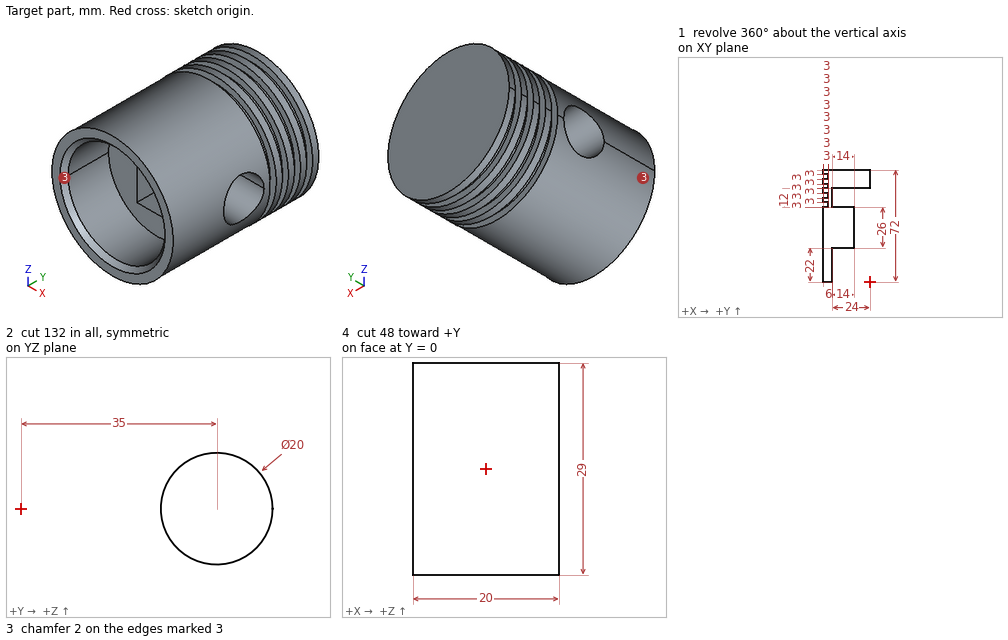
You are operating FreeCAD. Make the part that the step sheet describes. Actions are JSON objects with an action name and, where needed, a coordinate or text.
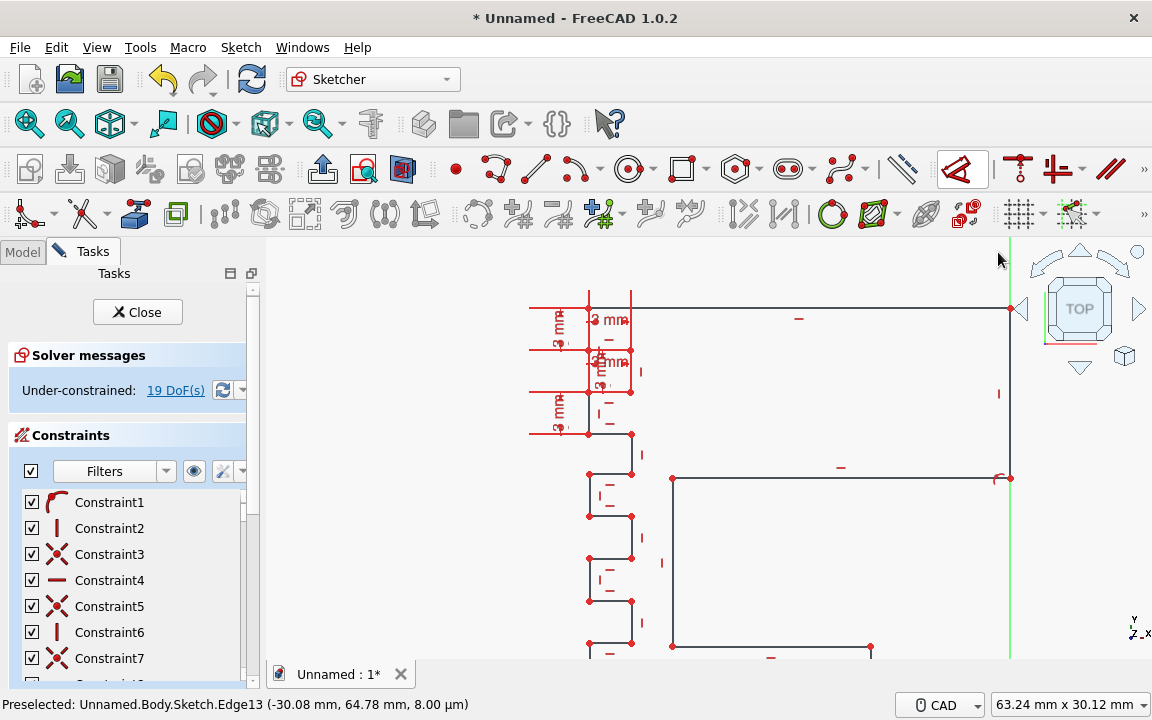
{"action": "left_click", "coordinate": [602, 434]}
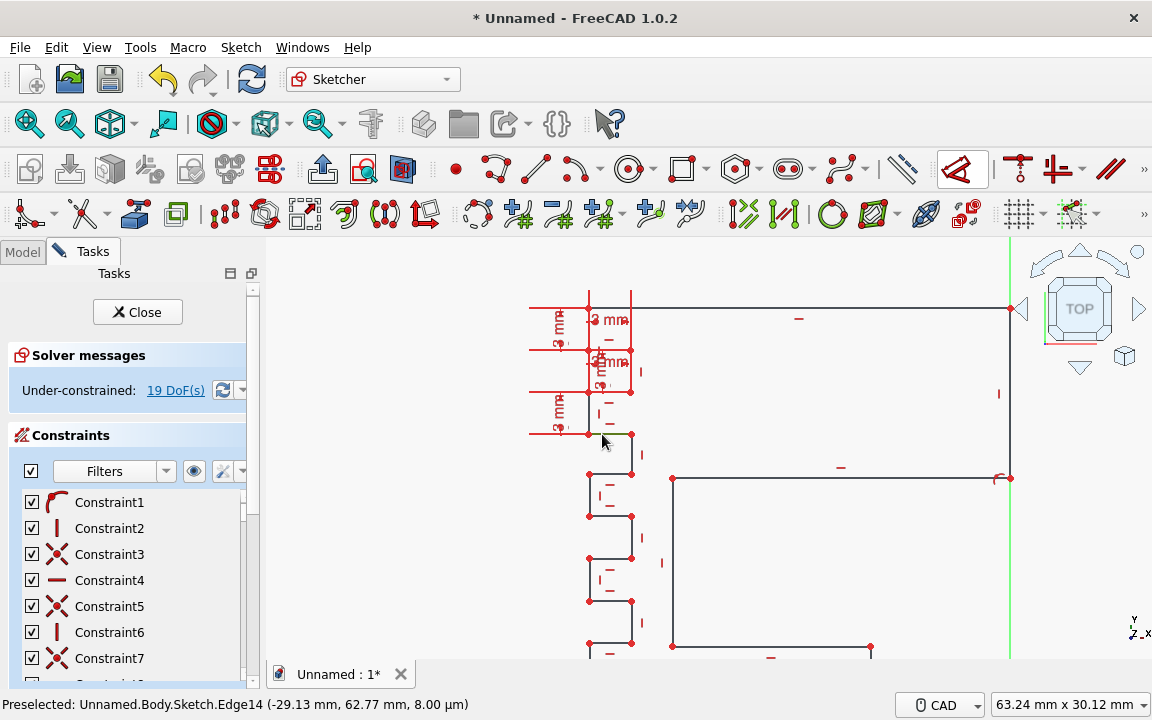
{"action": "left_click", "coordinate": [982, 170]}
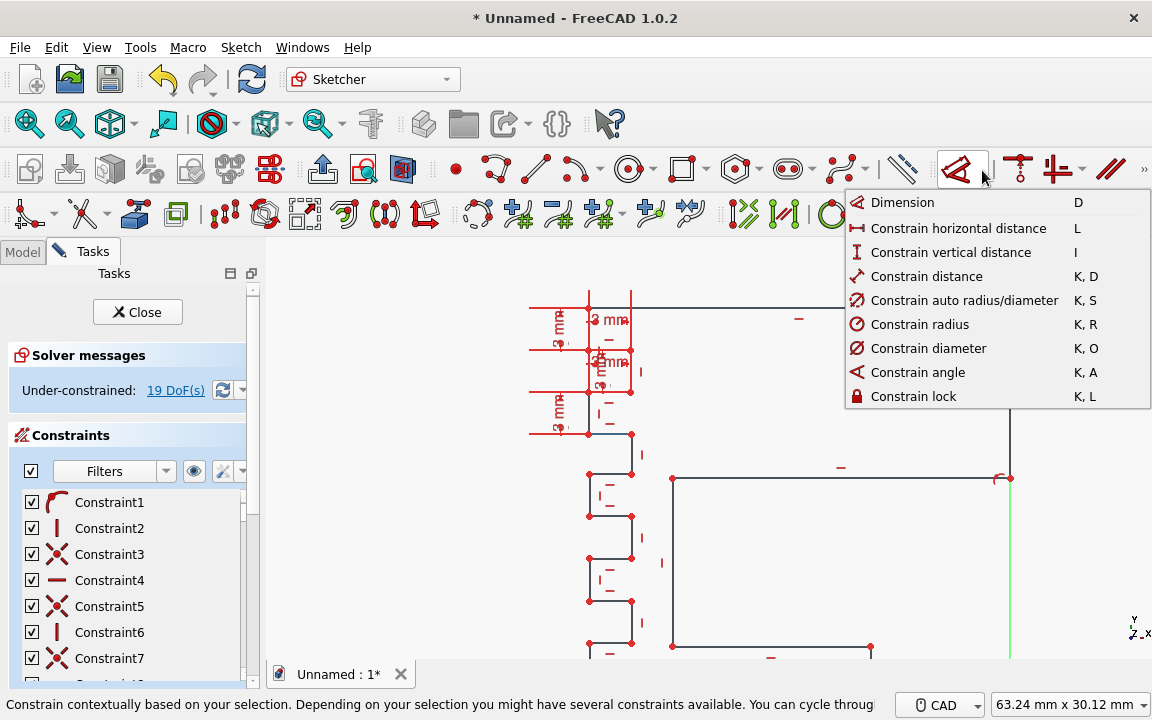
{"action": "left_click", "coordinate": [998, 228]}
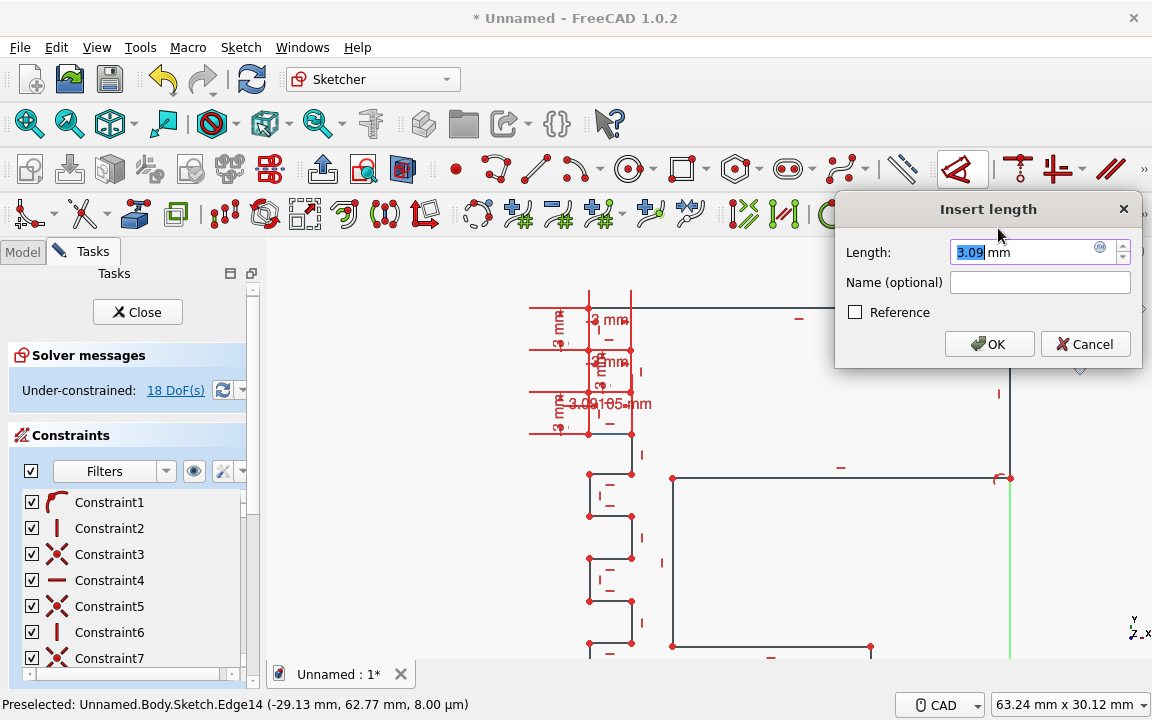
{"action": "type", "text": "3"}
{"action": "key", "text": "Return"}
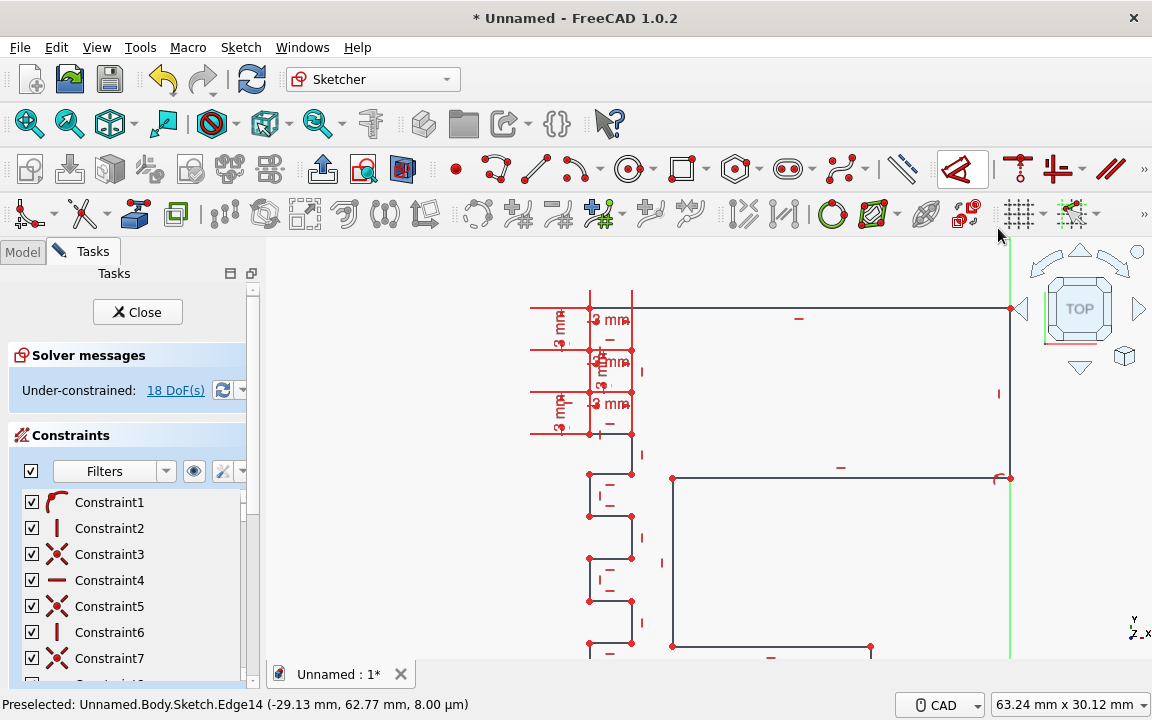
{"action": "left_click", "coordinate": [632, 446]}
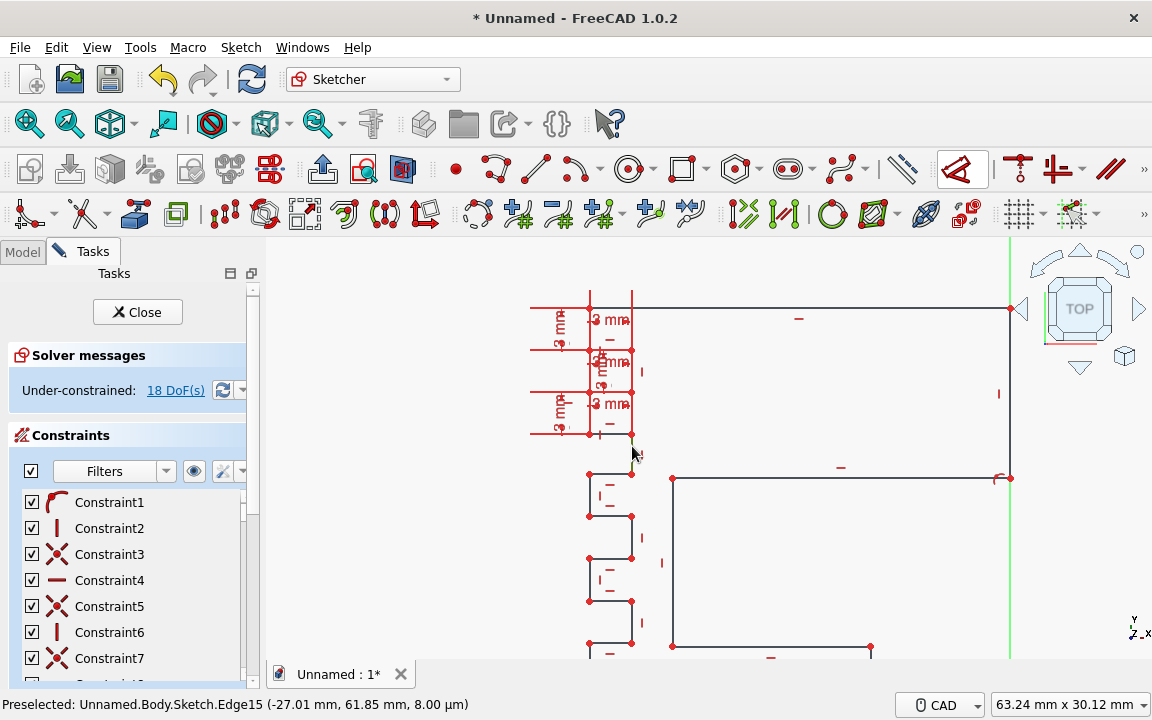
{"action": "left_click", "coordinate": [982, 170]}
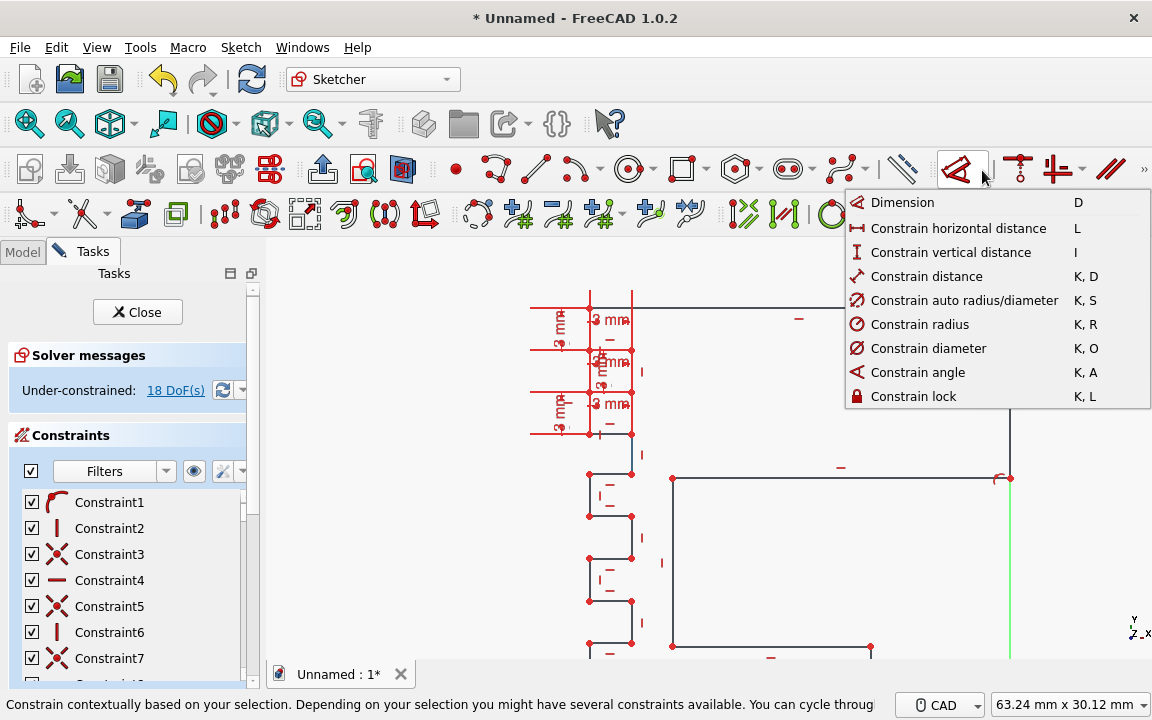
{"action": "left_click", "coordinate": [998, 252]}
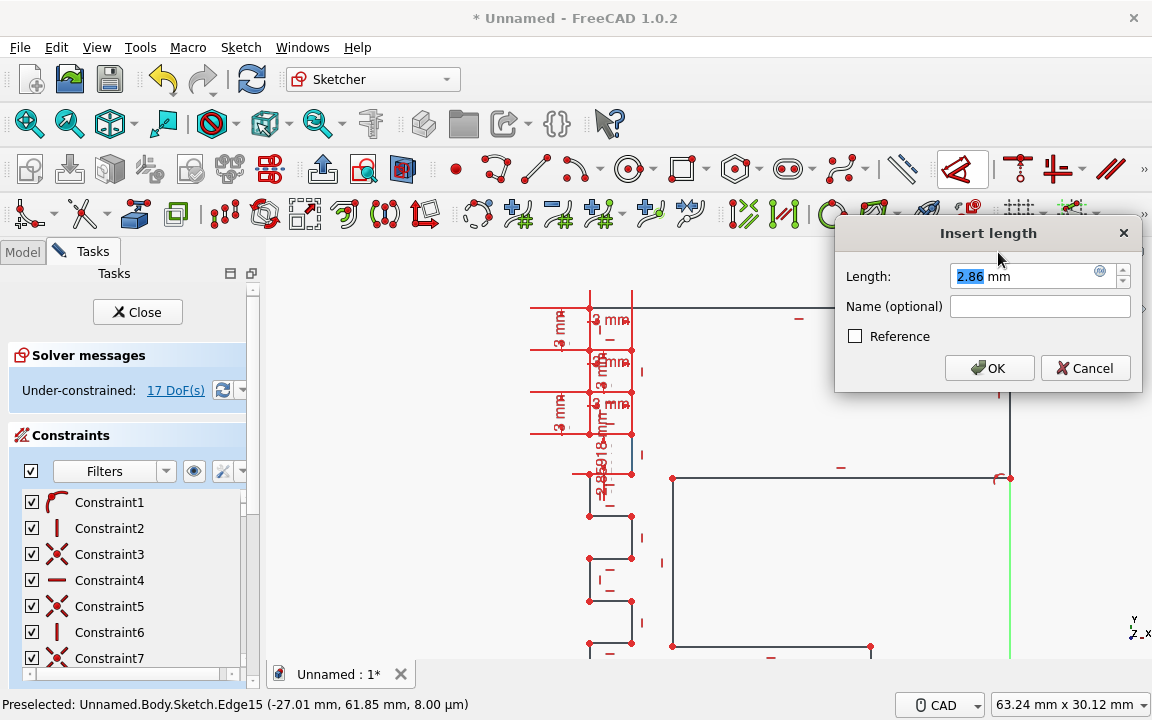
{"action": "type", "text": "3"}
{"action": "key", "text": "Return"}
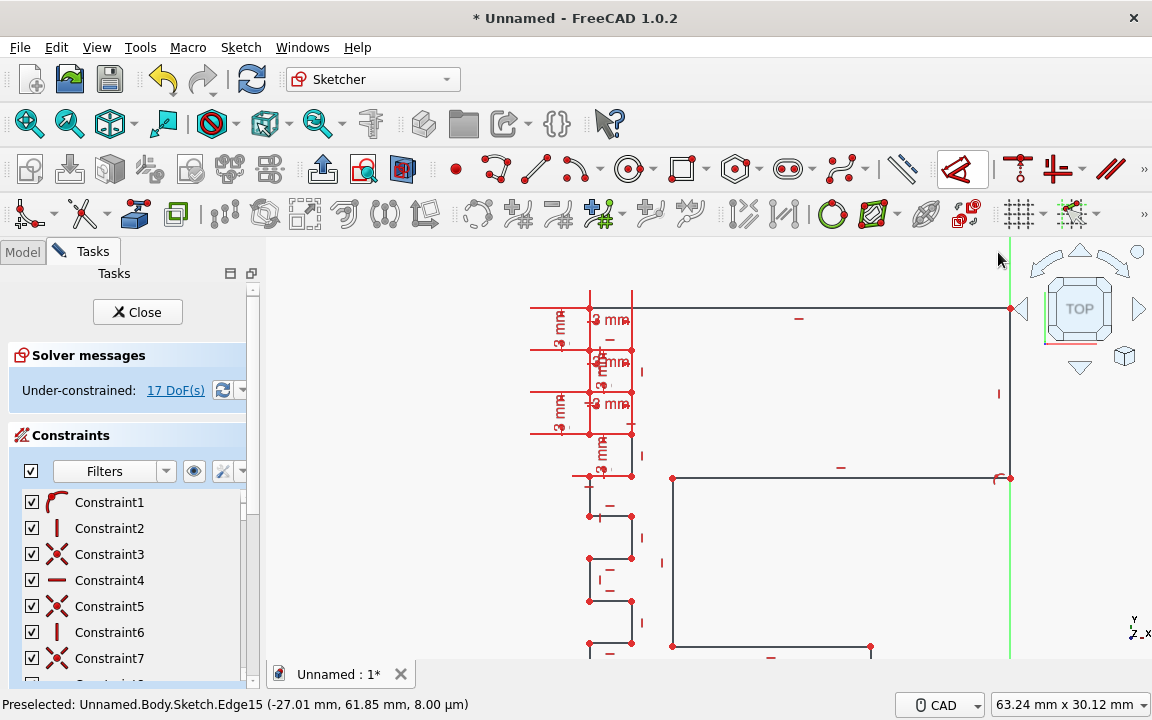
{"action": "left_click", "coordinate": [619, 476]}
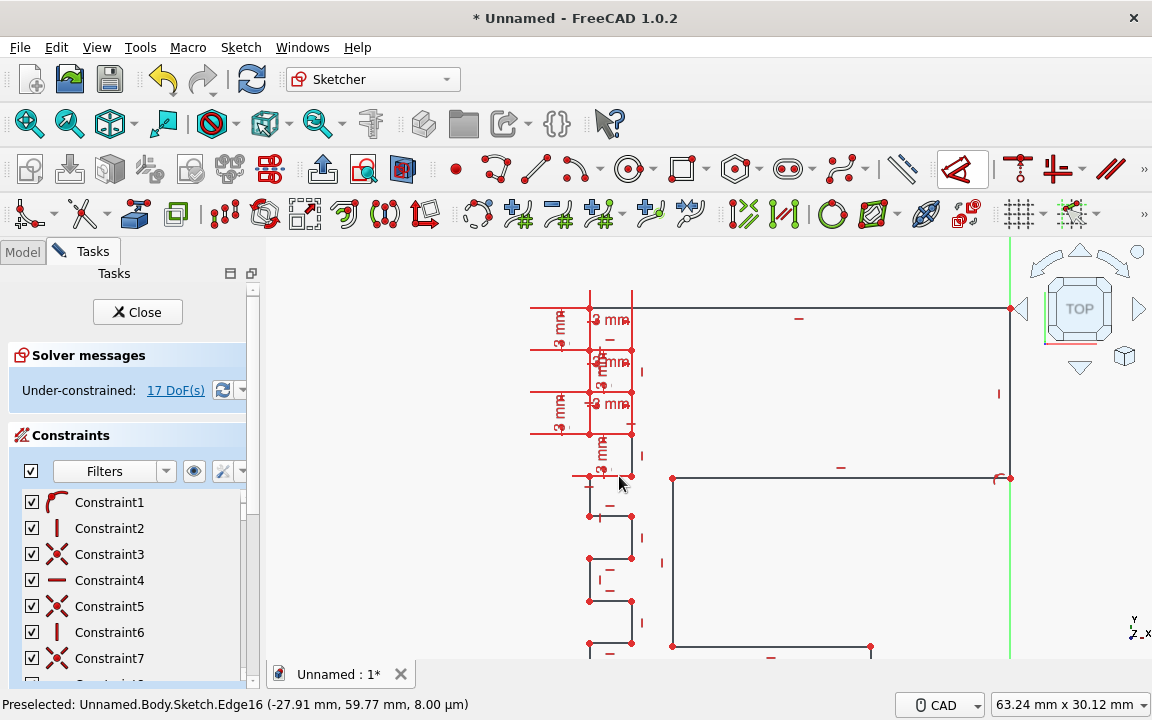
{"action": "key", "text": "l"}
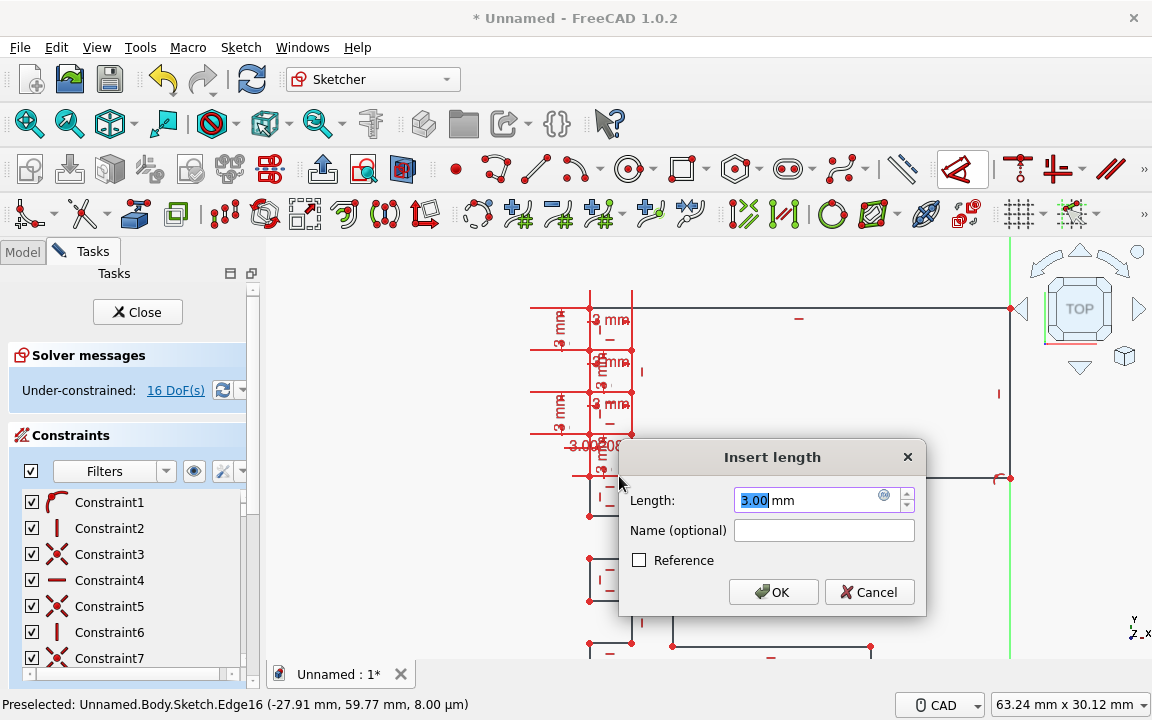
{"action": "type", "text": "3"}
{"action": "key", "text": "Return"}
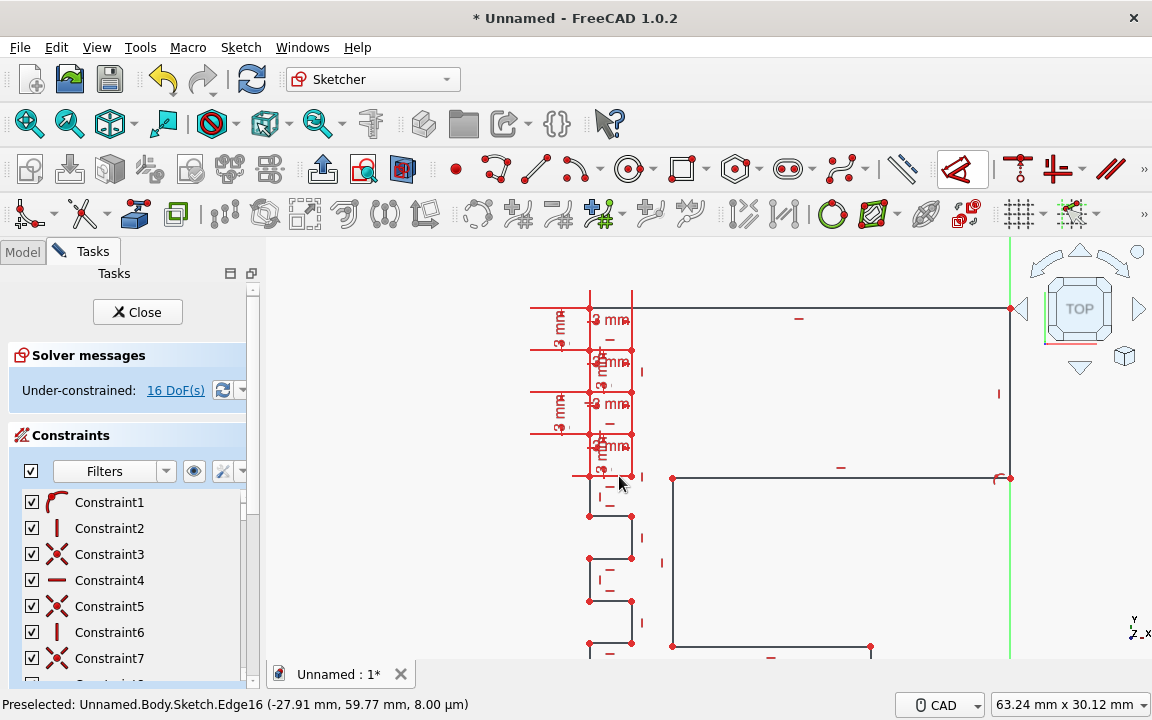
{"action": "left_click", "coordinate": [590, 488]}